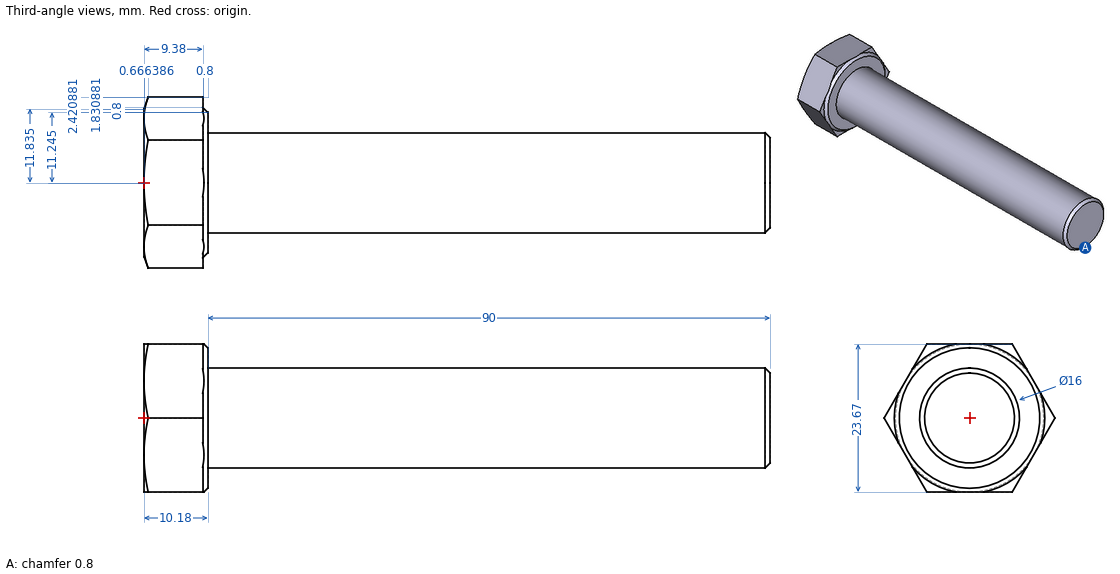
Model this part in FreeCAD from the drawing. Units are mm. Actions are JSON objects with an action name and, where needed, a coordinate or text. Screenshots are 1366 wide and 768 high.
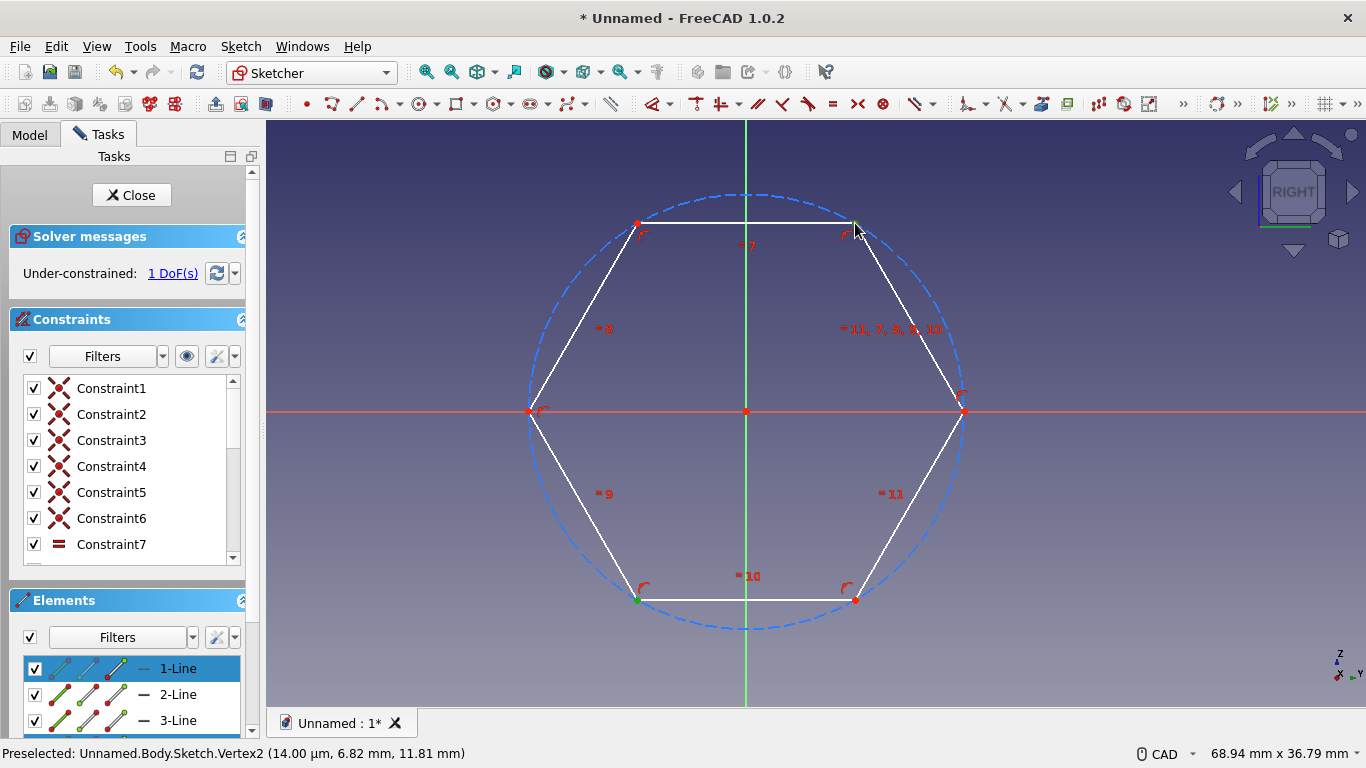
{"action": "left_click", "coordinate": [670, 104]}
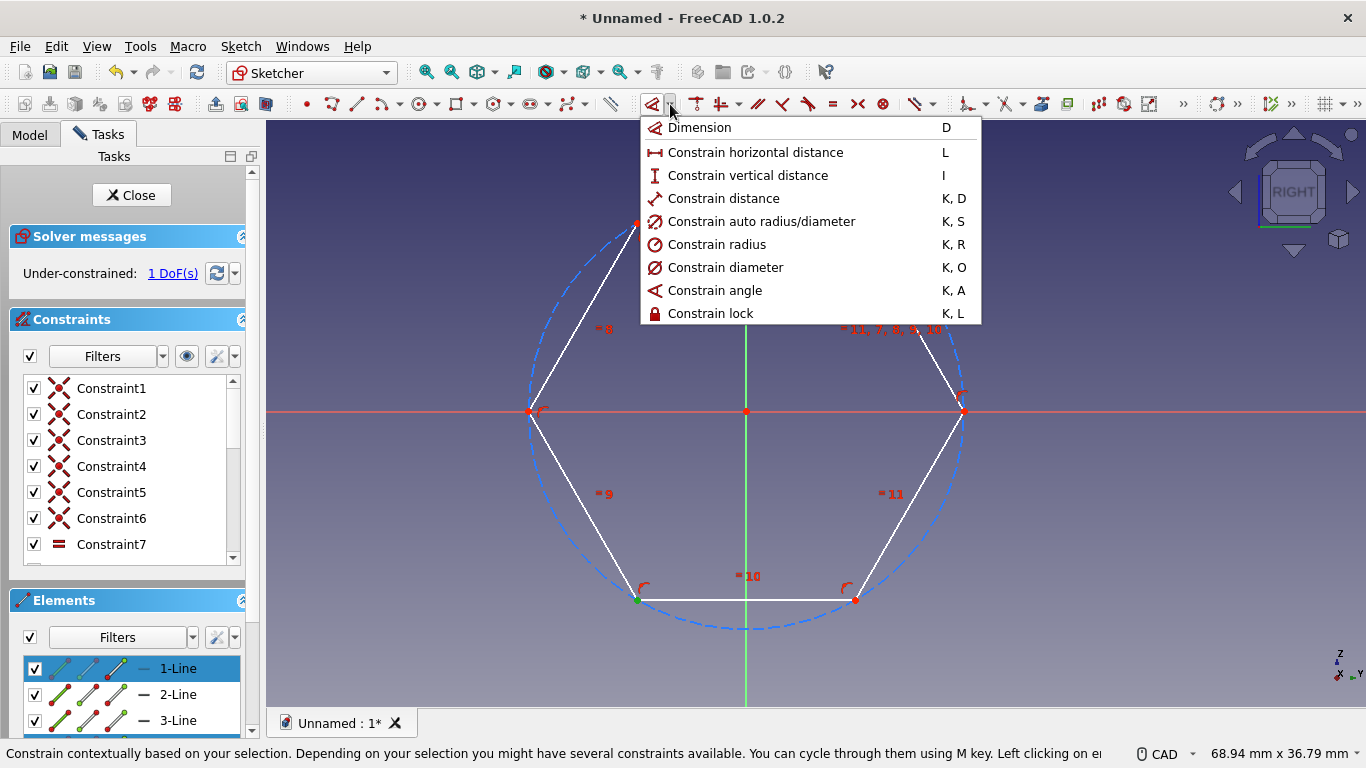
{"action": "left_click", "coordinate": [811, 176]}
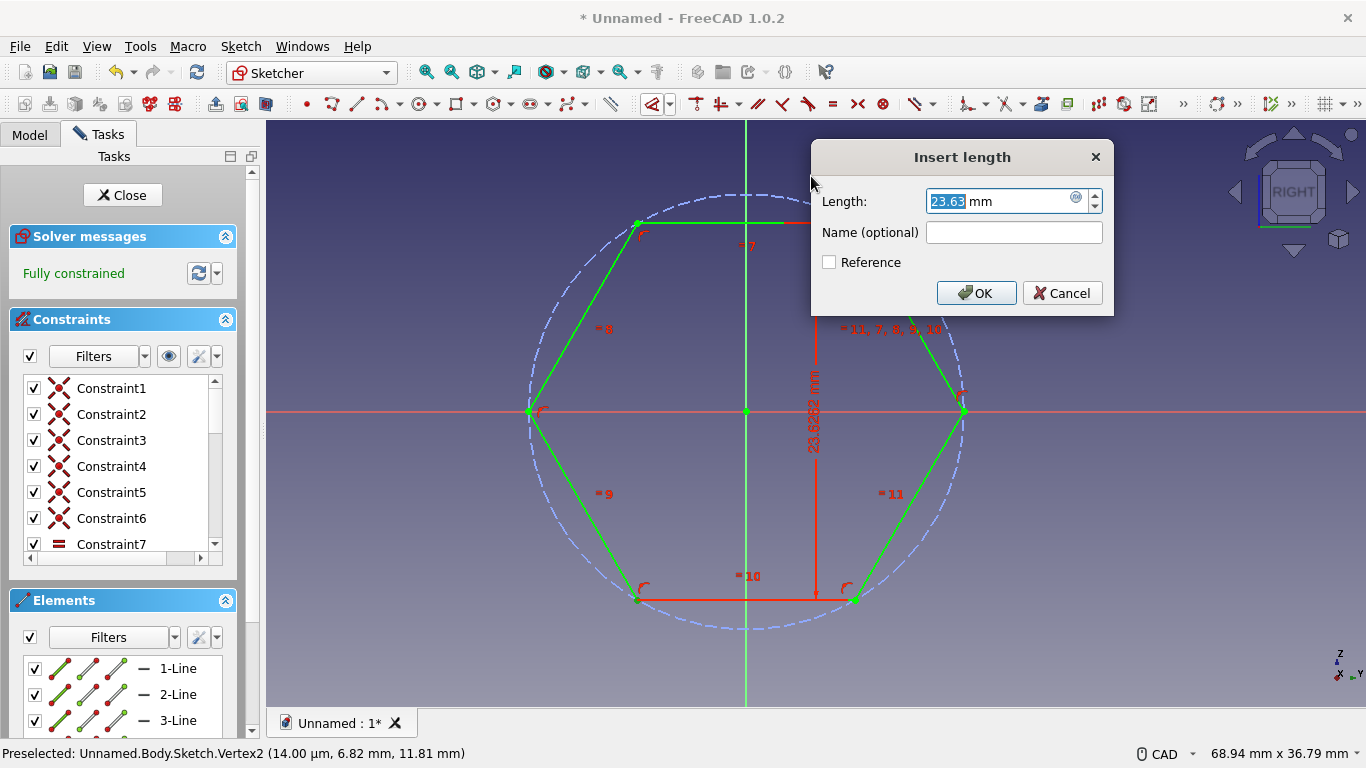
{"action": "type", "text": "23.67"}
{"action": "key", "text": "Return"}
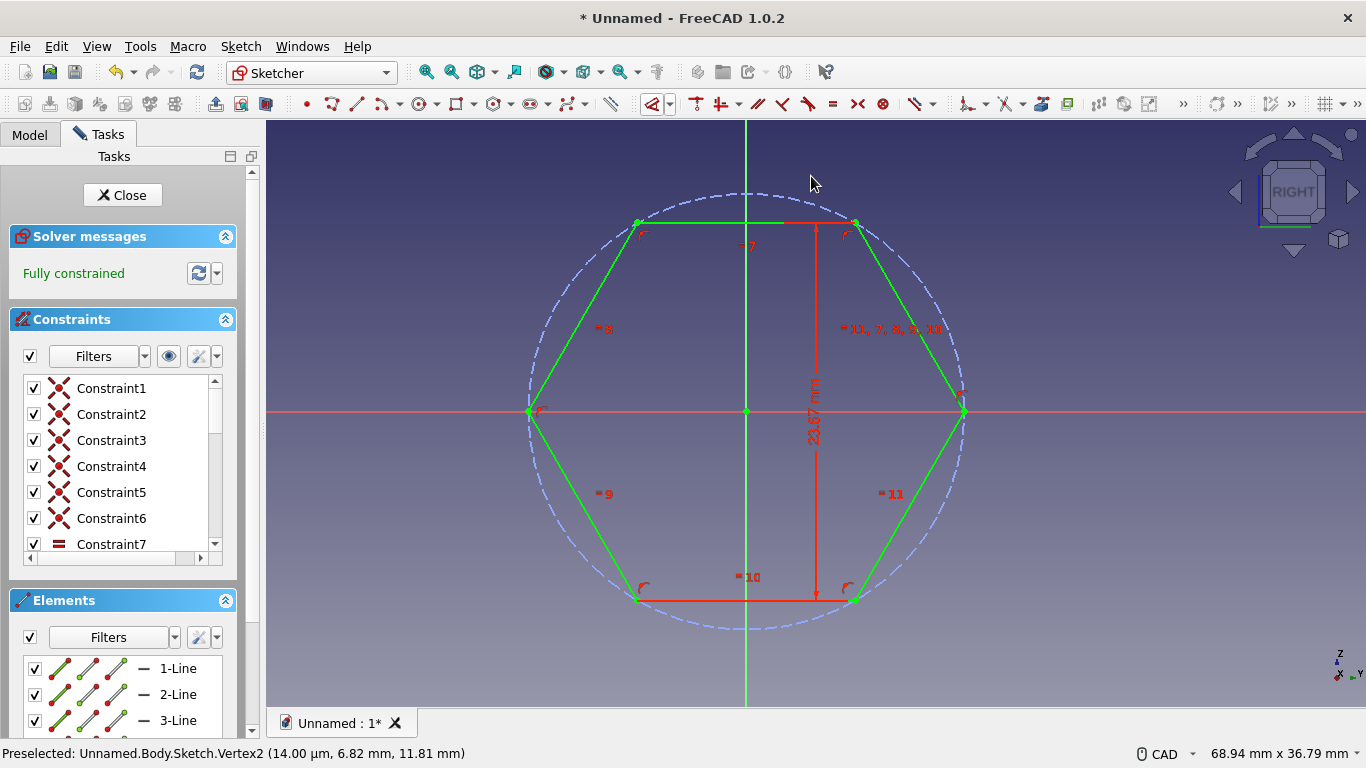
{"action": "left_click", "coordinate": [123, 195]}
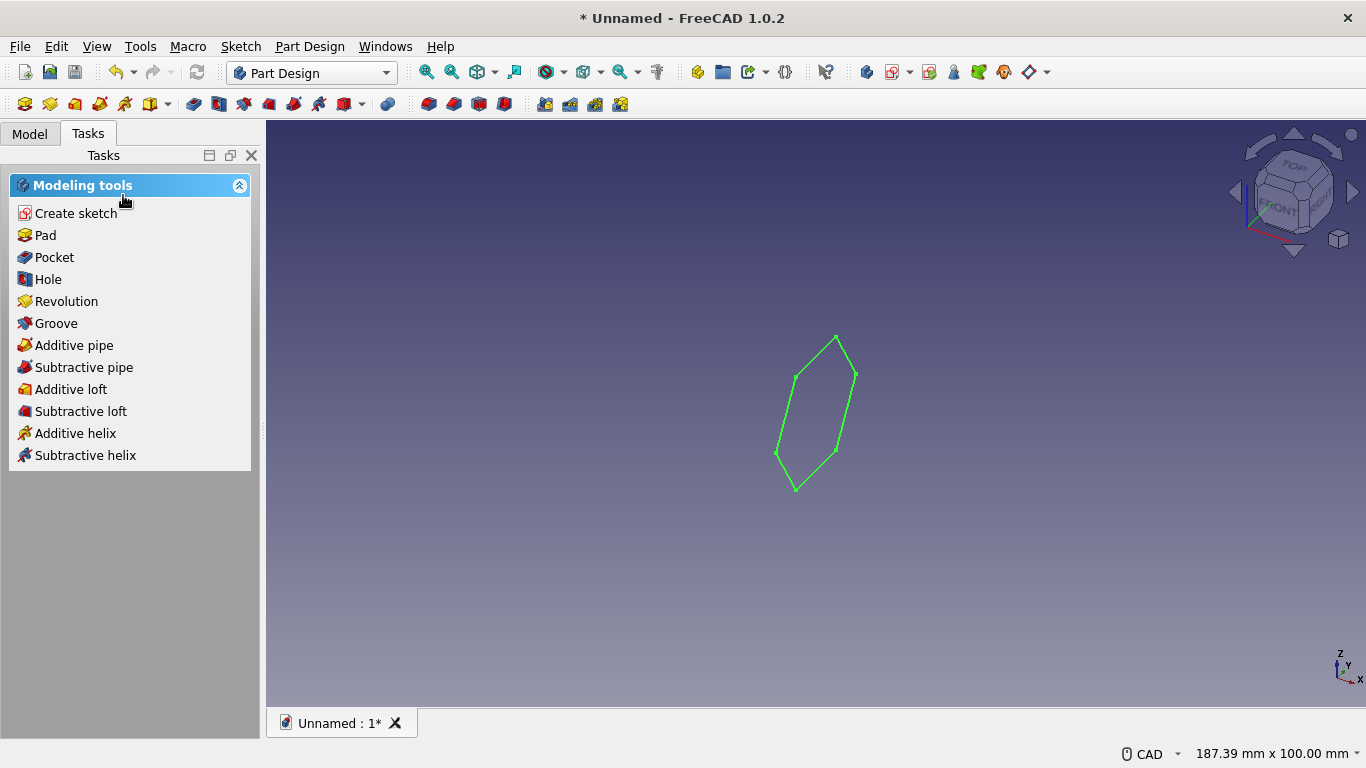
{"action": "left_click", "coordinate": [25, 104]}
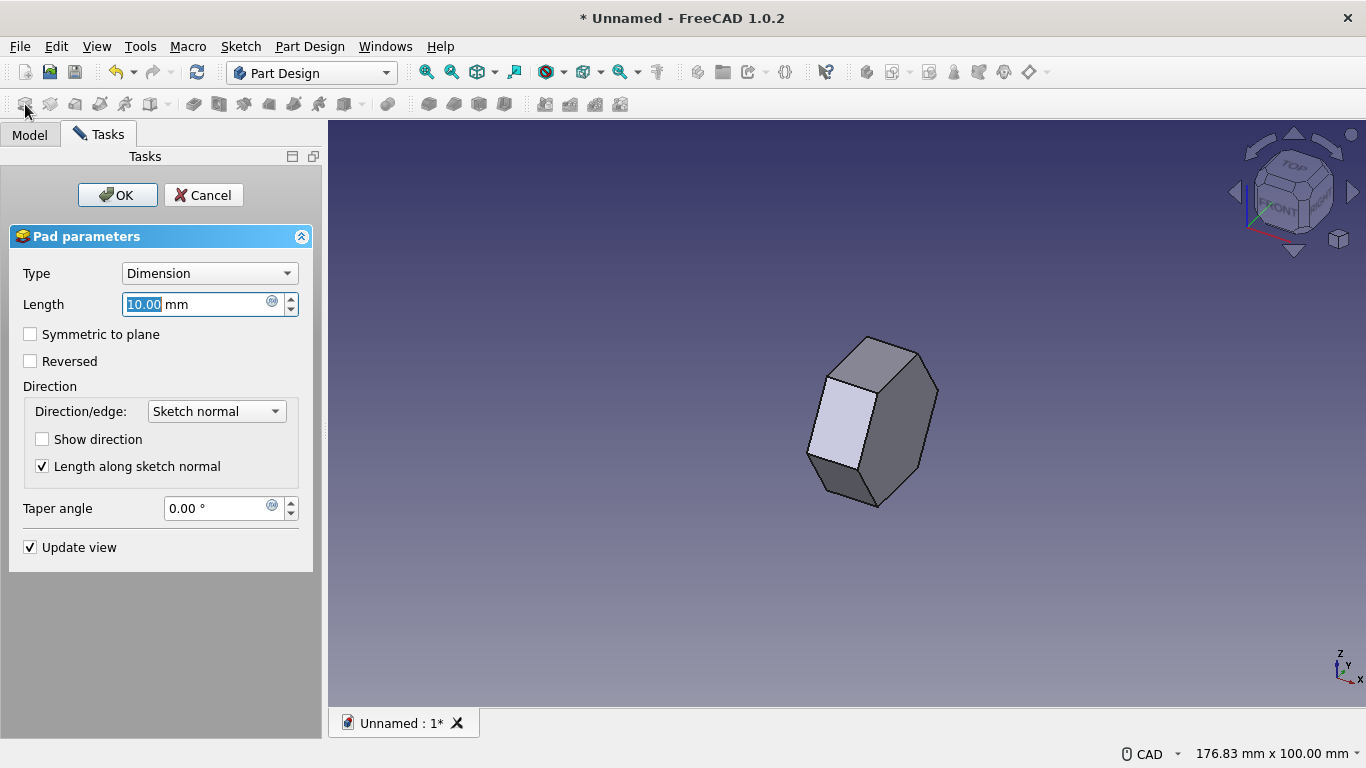
{"action": "type", "text": "10.18"}
{"action": "key", "text": "Tab"}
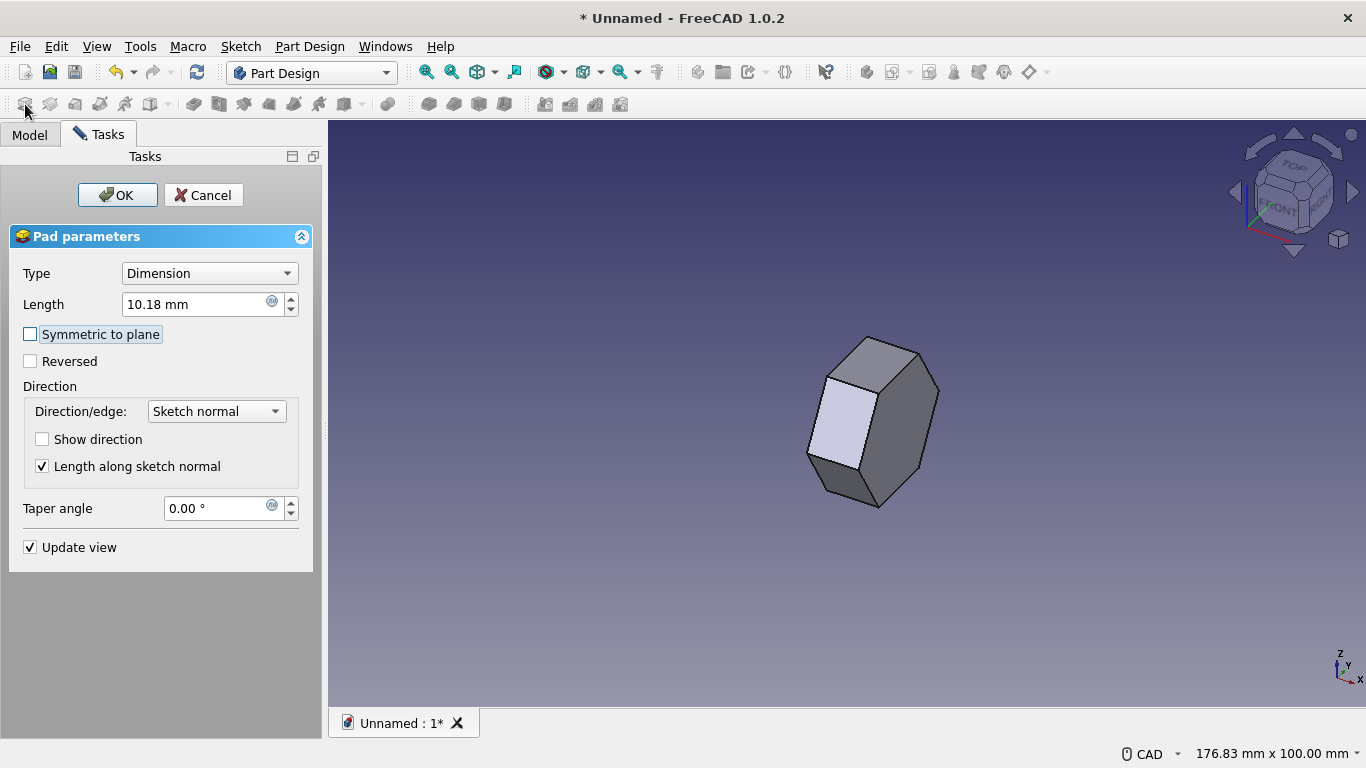
{"action": "left_click", "coordinate": [118, 195]}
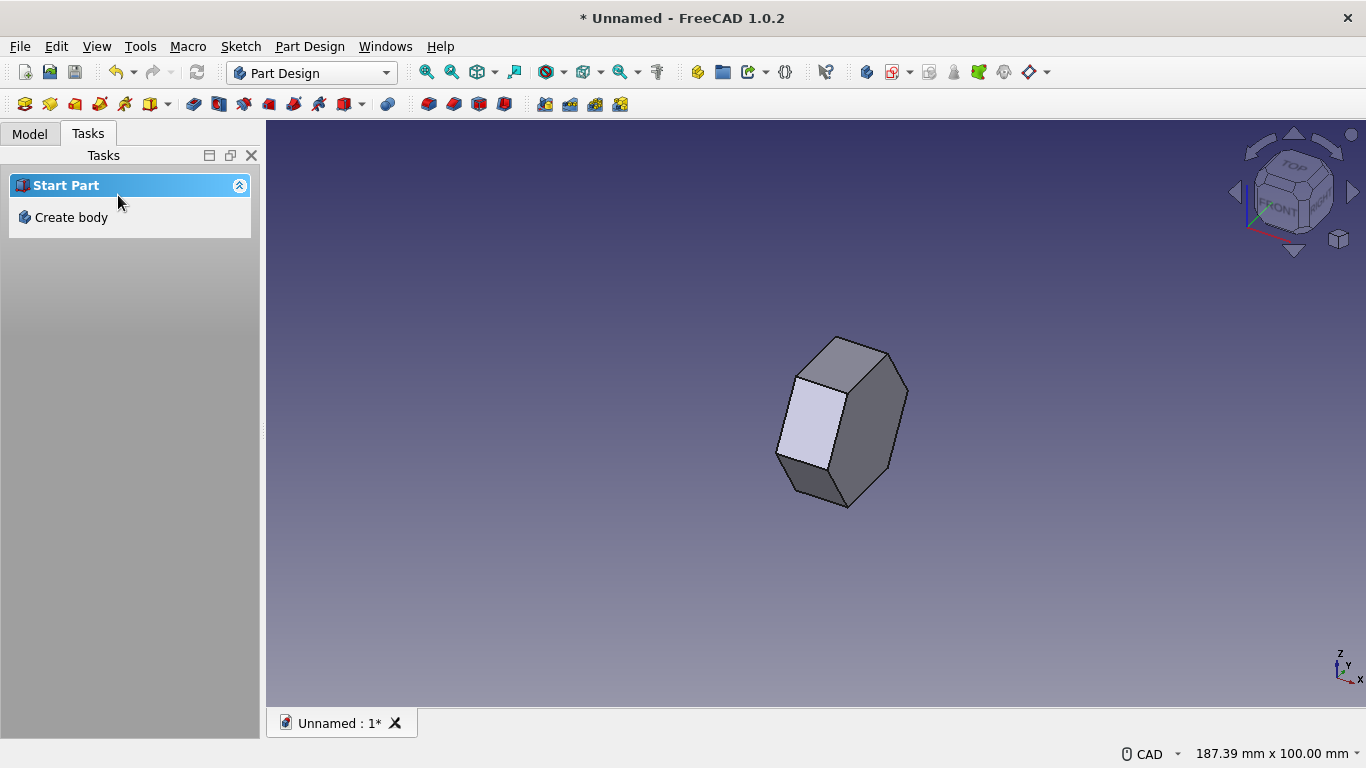
{"action": "key", "text": "v f"}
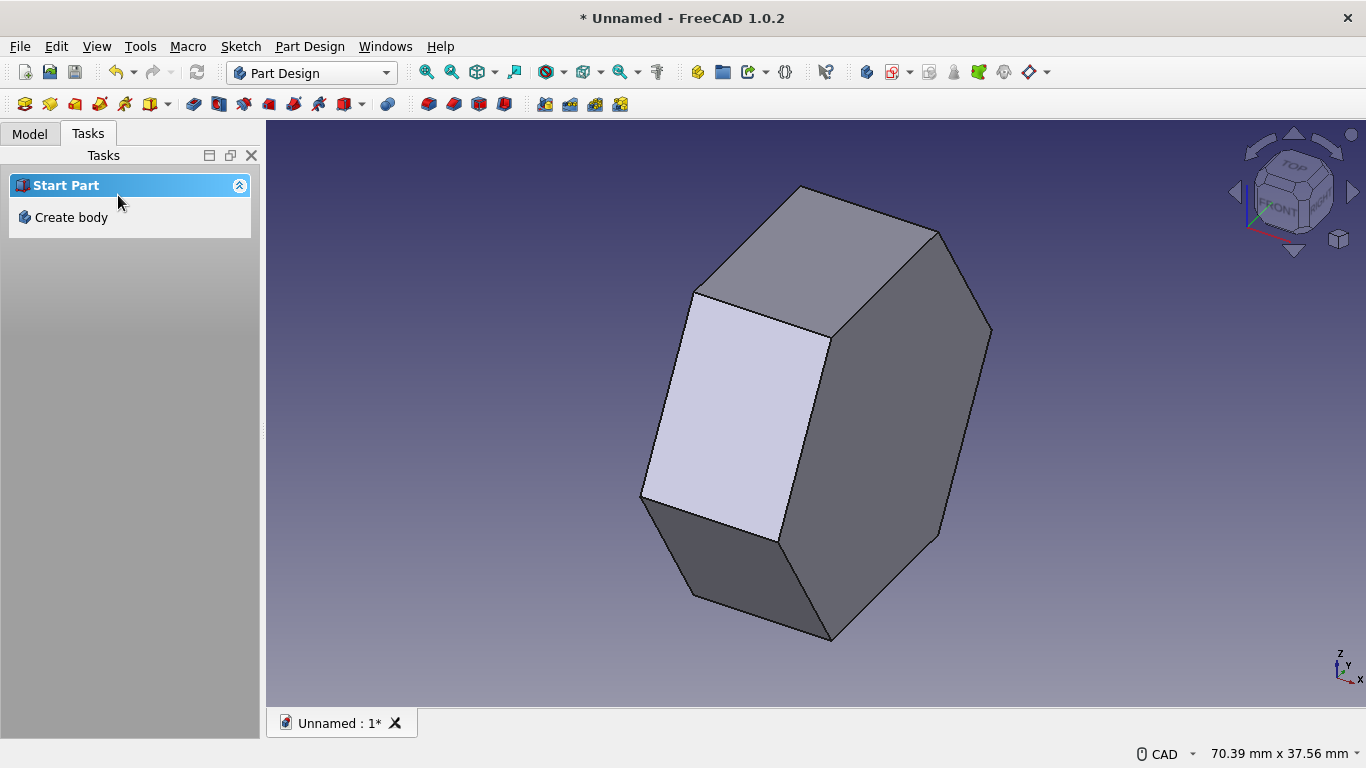
{"action": "left_click", "coordinate": [892, 72]}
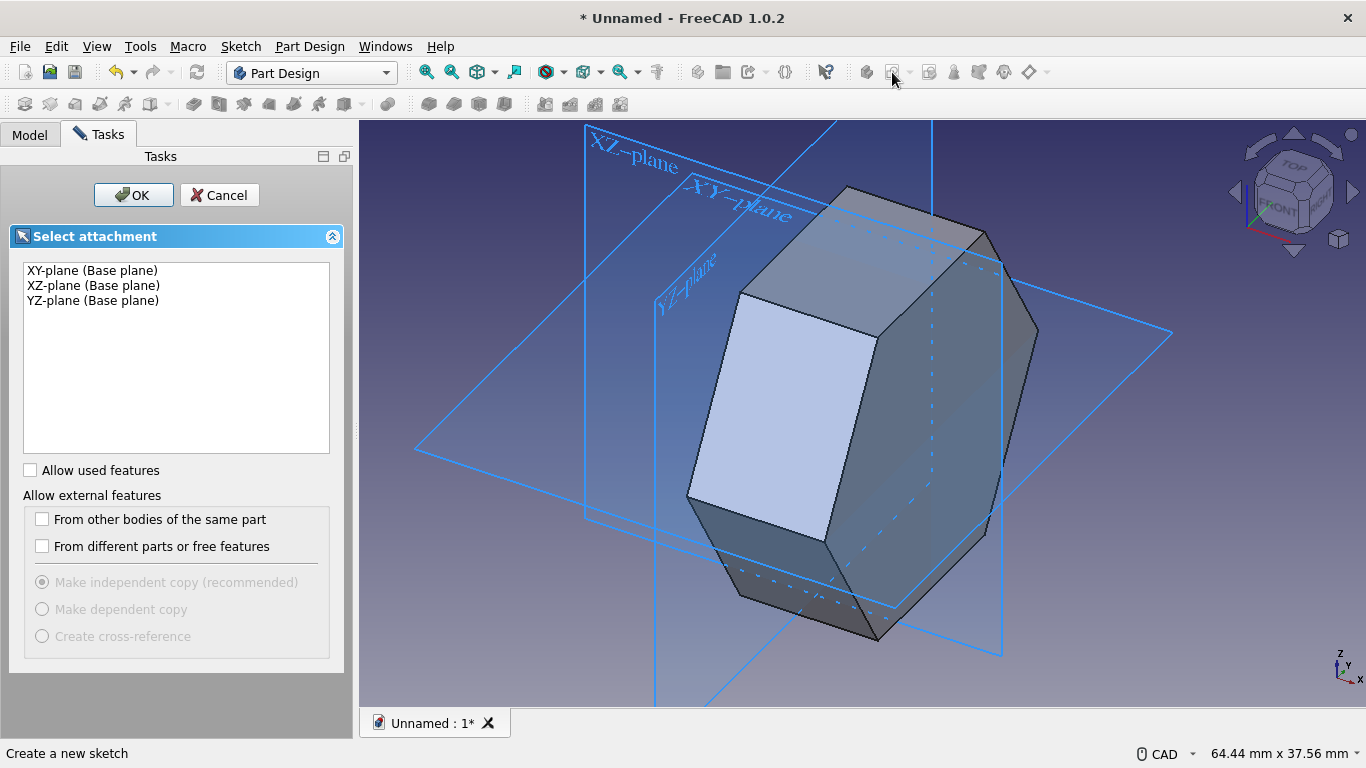
{"action": "left_click", "coordinate": [84, 270]}